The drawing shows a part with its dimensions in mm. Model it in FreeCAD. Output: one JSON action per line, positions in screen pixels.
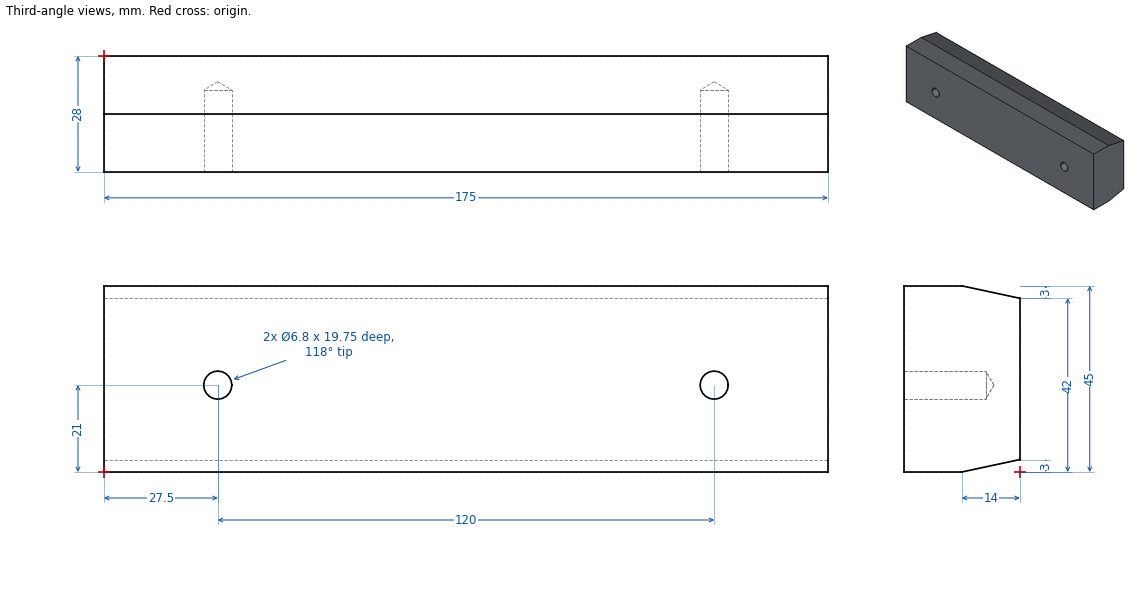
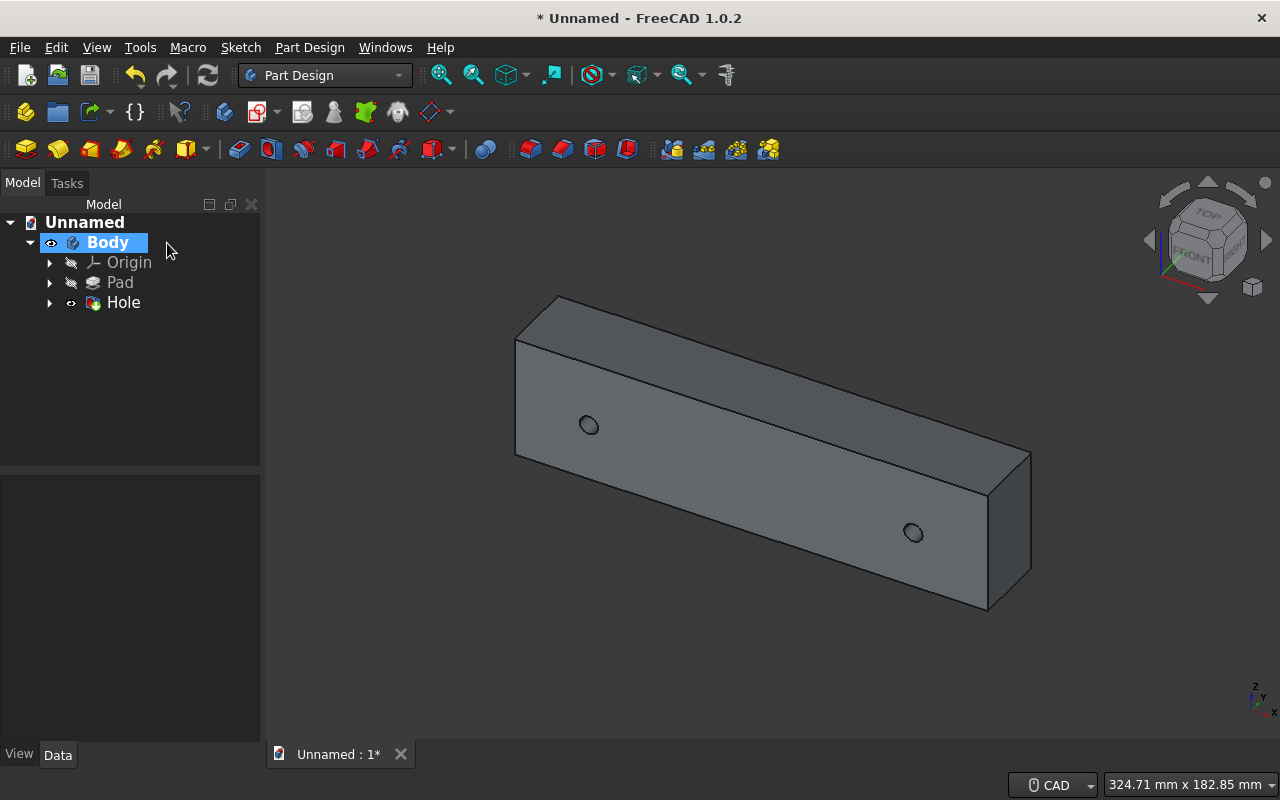
{"action": "key", "text": "6"}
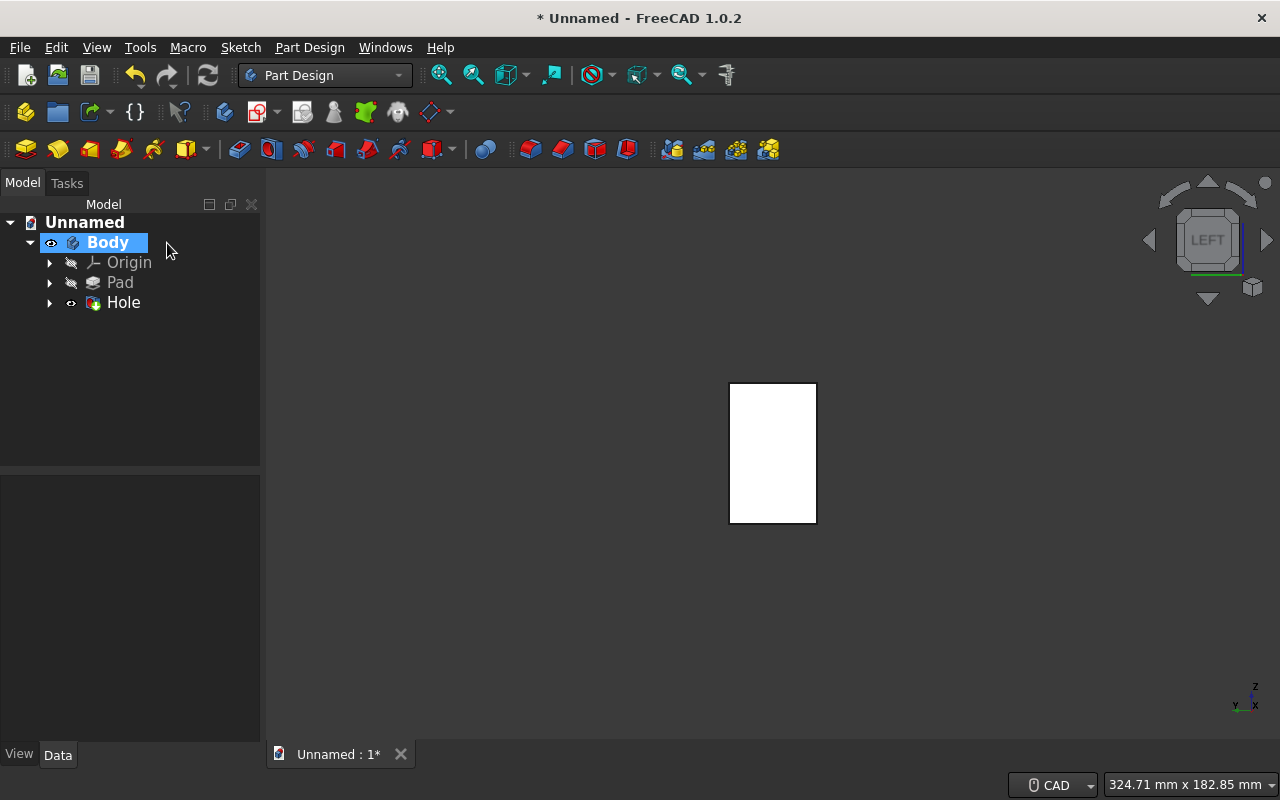
{"action": "left_click", "coordinate": [442, 76]}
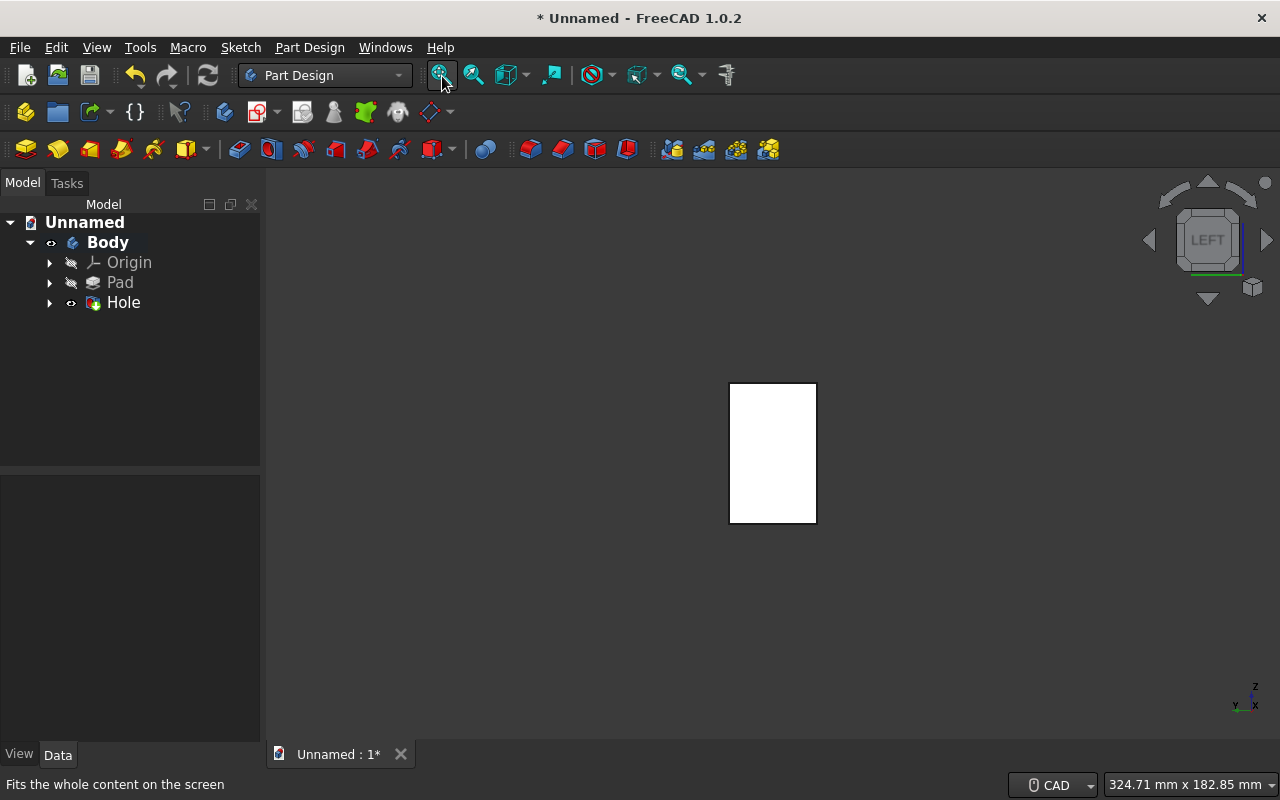
{"action": "left_click", "coordinate": [773, 432]}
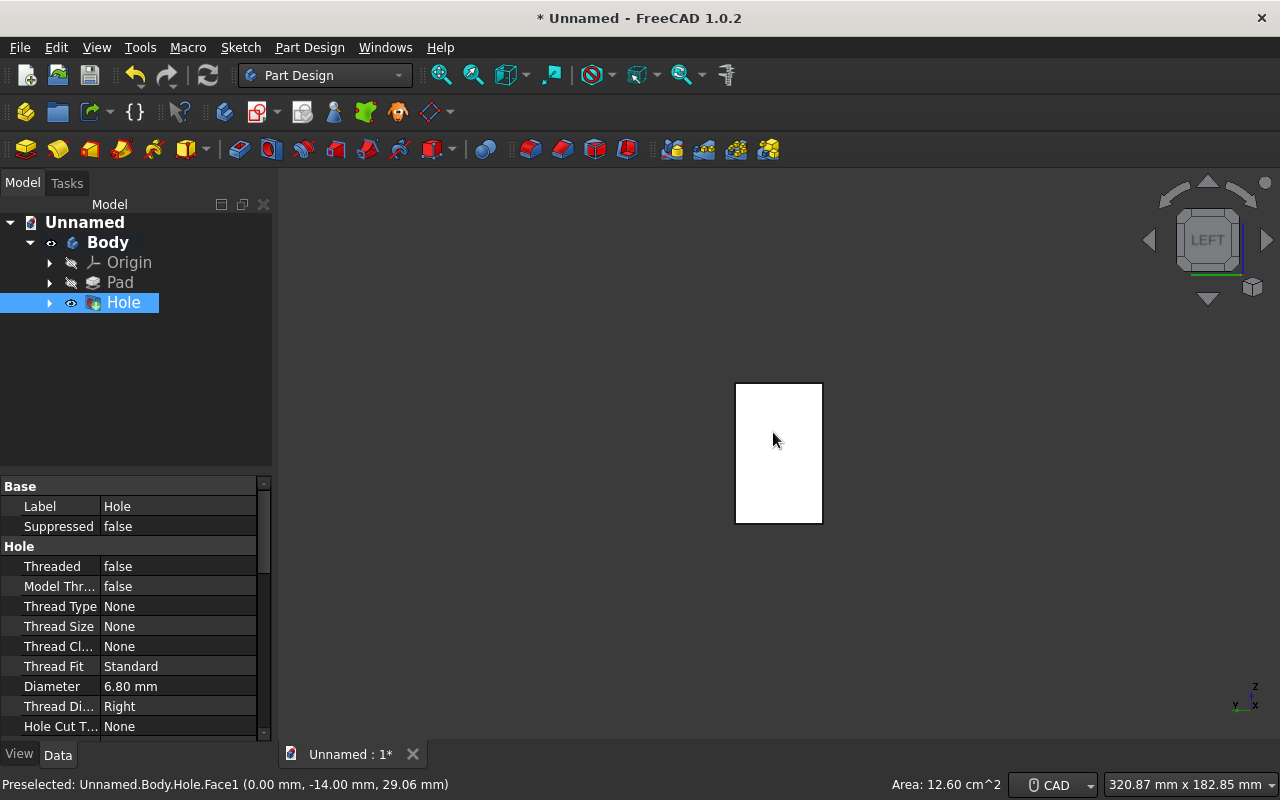
{"action": "left_click", "coordinate": [258, 112]}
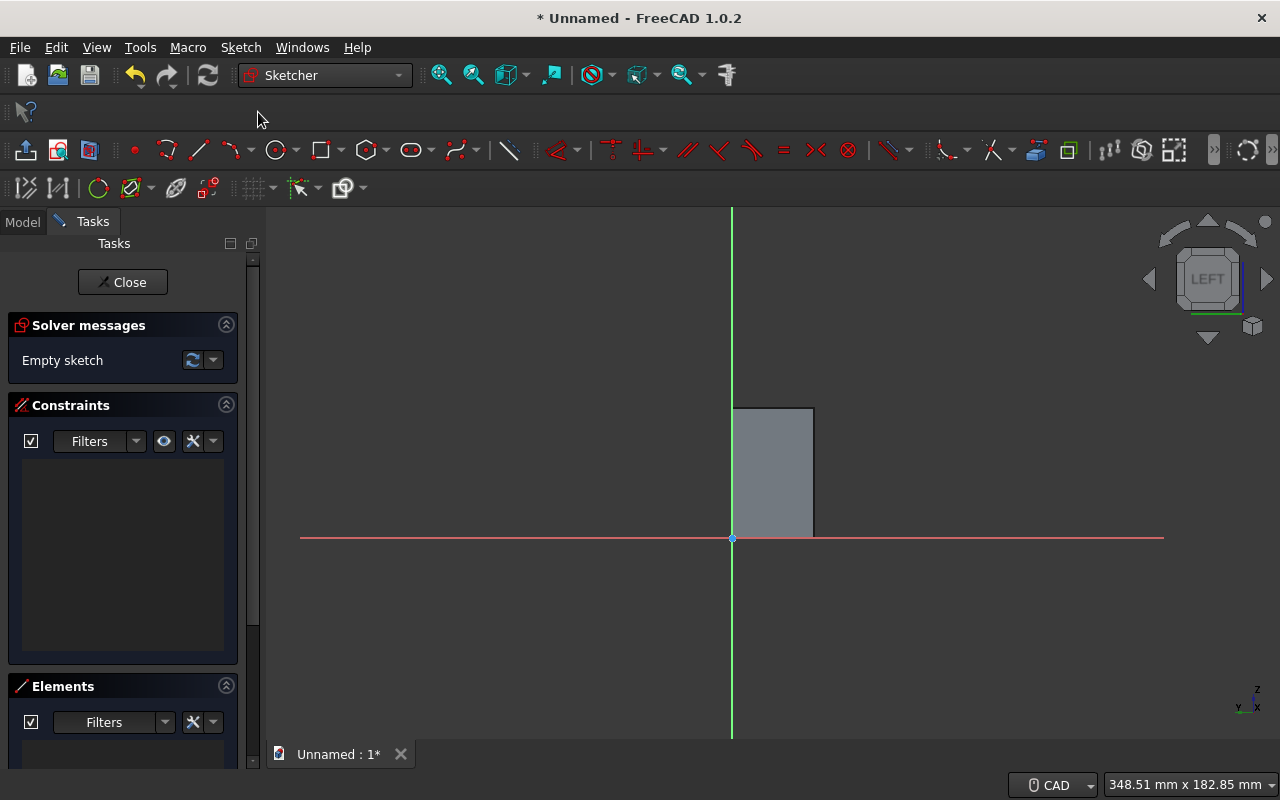
{"action": "scroll", "coordinate": [781, 473], "scroll_direction": "up", "scroll_amount": 5}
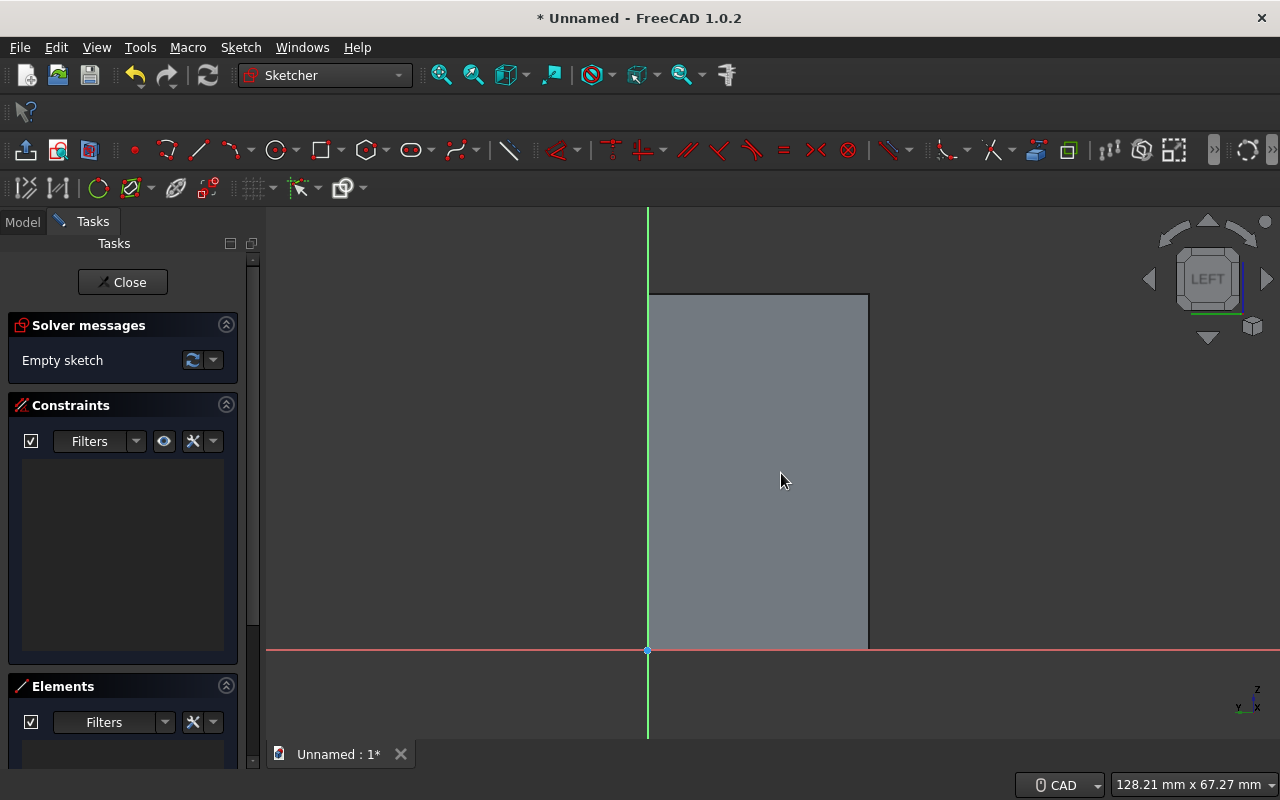
{"action": "left_click", "coordinate": [168, 150]}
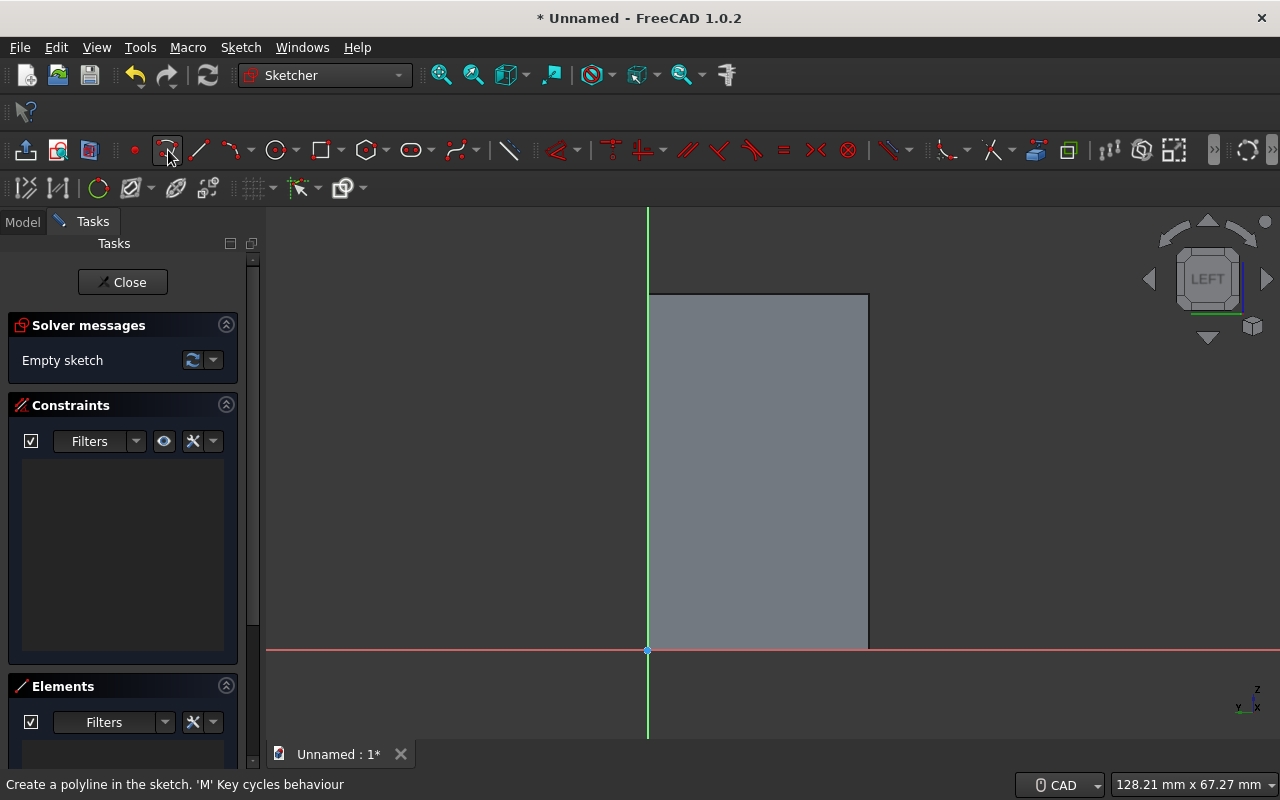
{"action": "left_click", "coordinate": [648, 650]}
{"action": "left_click", "coordinate": [758, 641]}
{"action": "left_click", "coordinate": [657, 626]}
{"action": "left_click", "coordinate": [648, 650]}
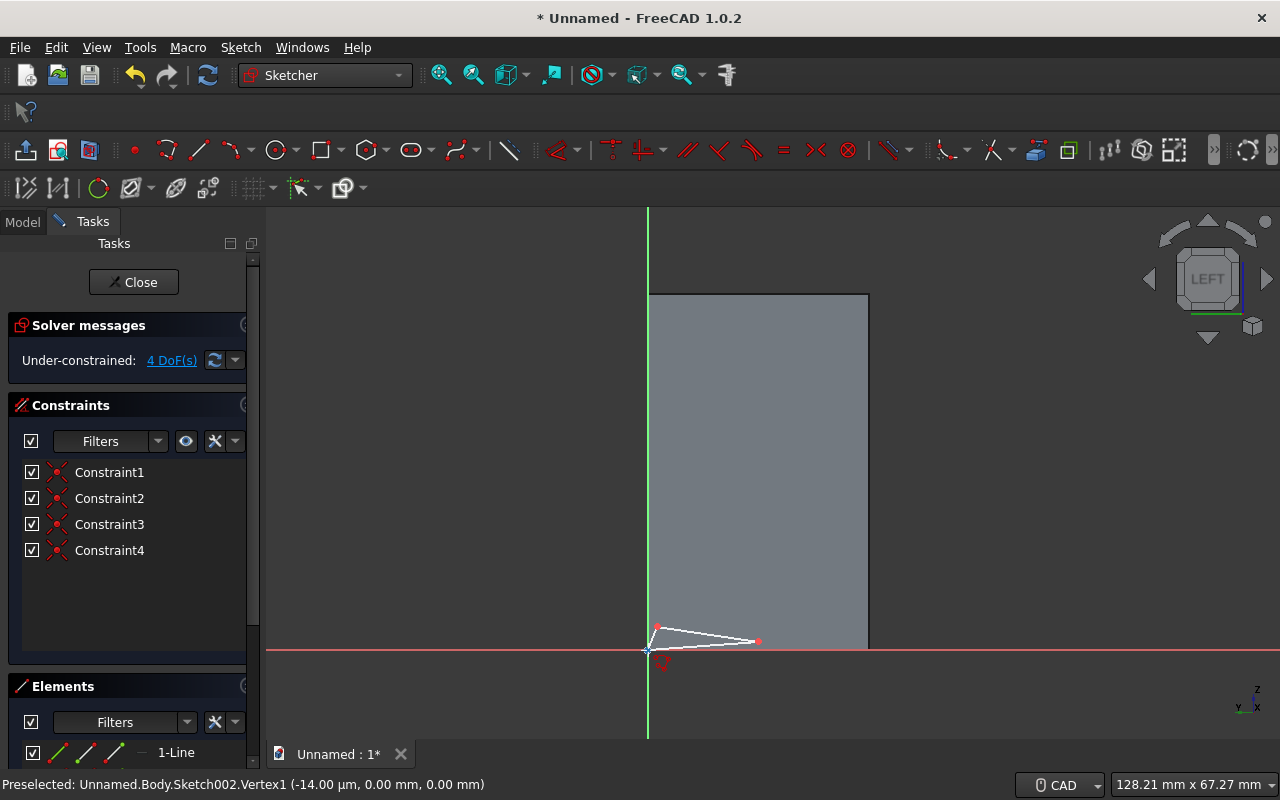
{"action": "left_click", "coordinate": [648, 318]}
{"action": "left_click", "coordinate": [758, 294]}
{"action": "left_click", "coordinate": [657, 294]}
{"action": "left_click", "coordinate": [648, 319]}
{"action": "key", "text": "Escape"}
{"action": "key", "text": "Escape"}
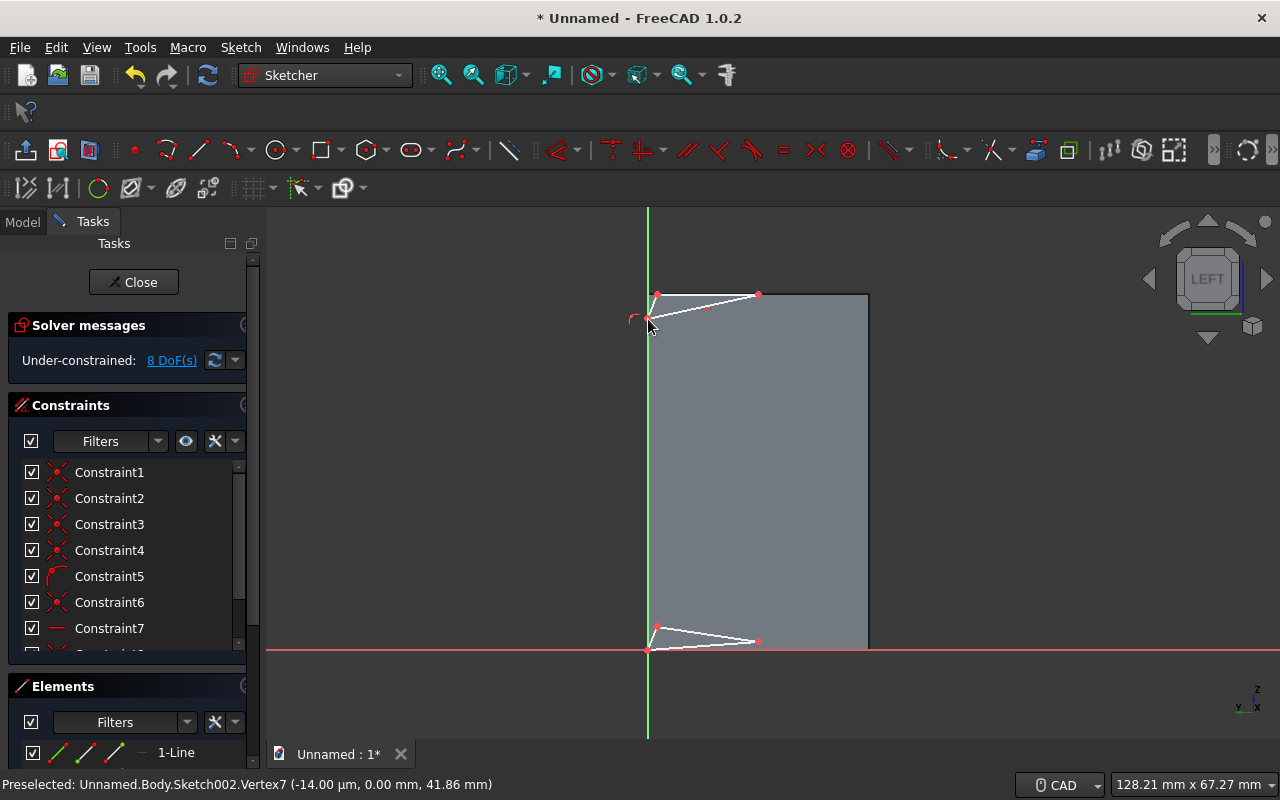
{"action": "left_click", "coordinate": [681, 648]}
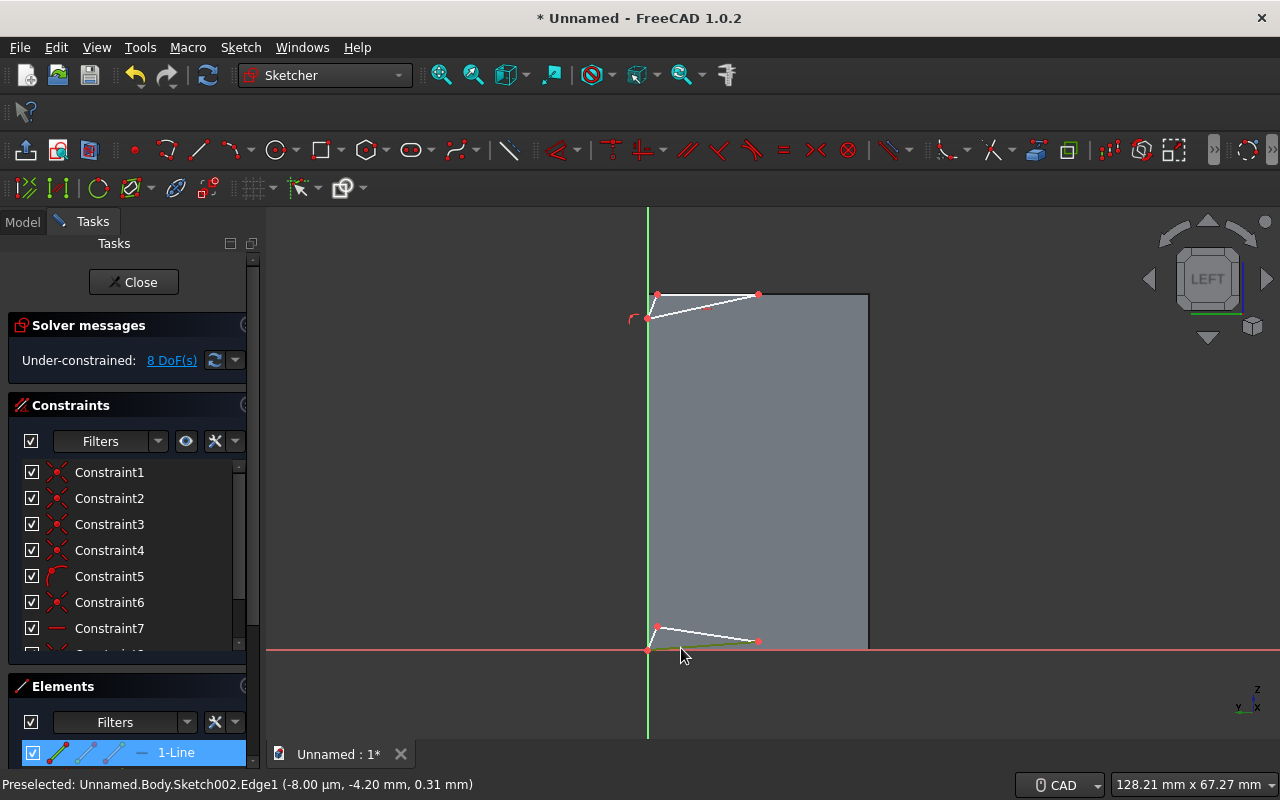
{"action": "key", "text": "h"}